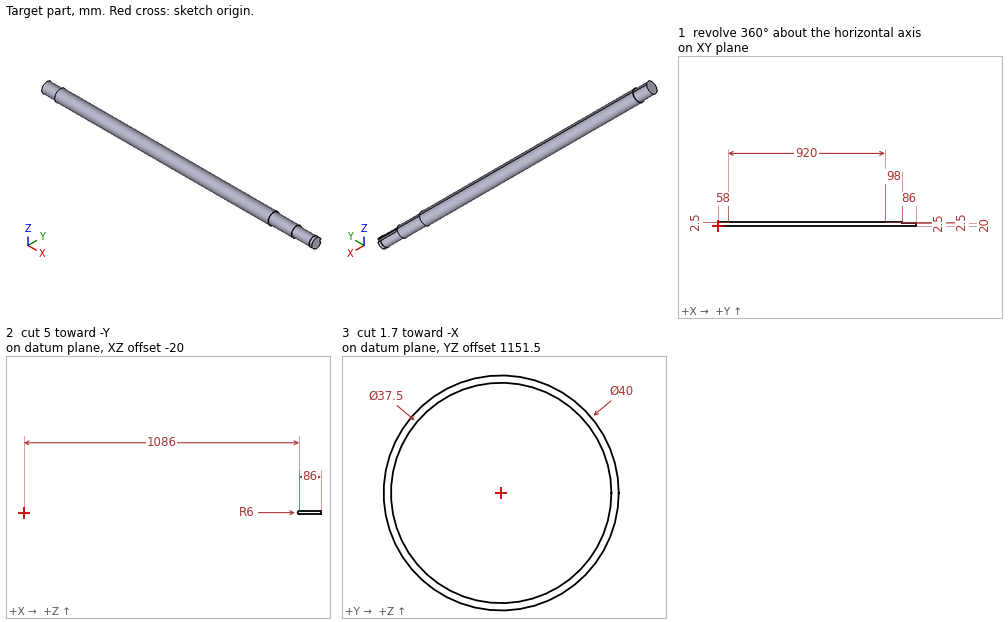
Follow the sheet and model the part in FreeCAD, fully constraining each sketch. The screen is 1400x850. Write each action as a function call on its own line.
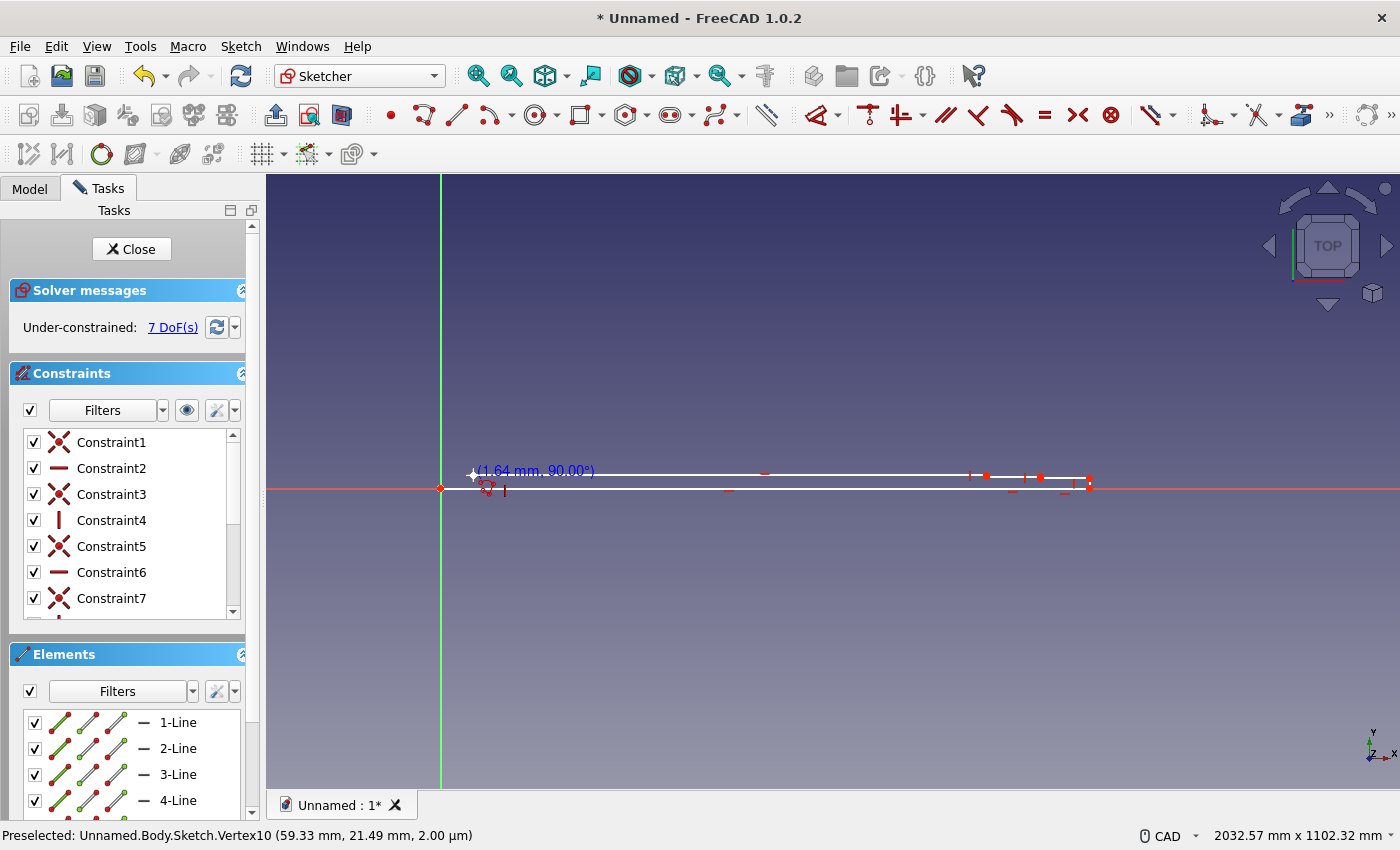
scroll(473, 476, up, 13)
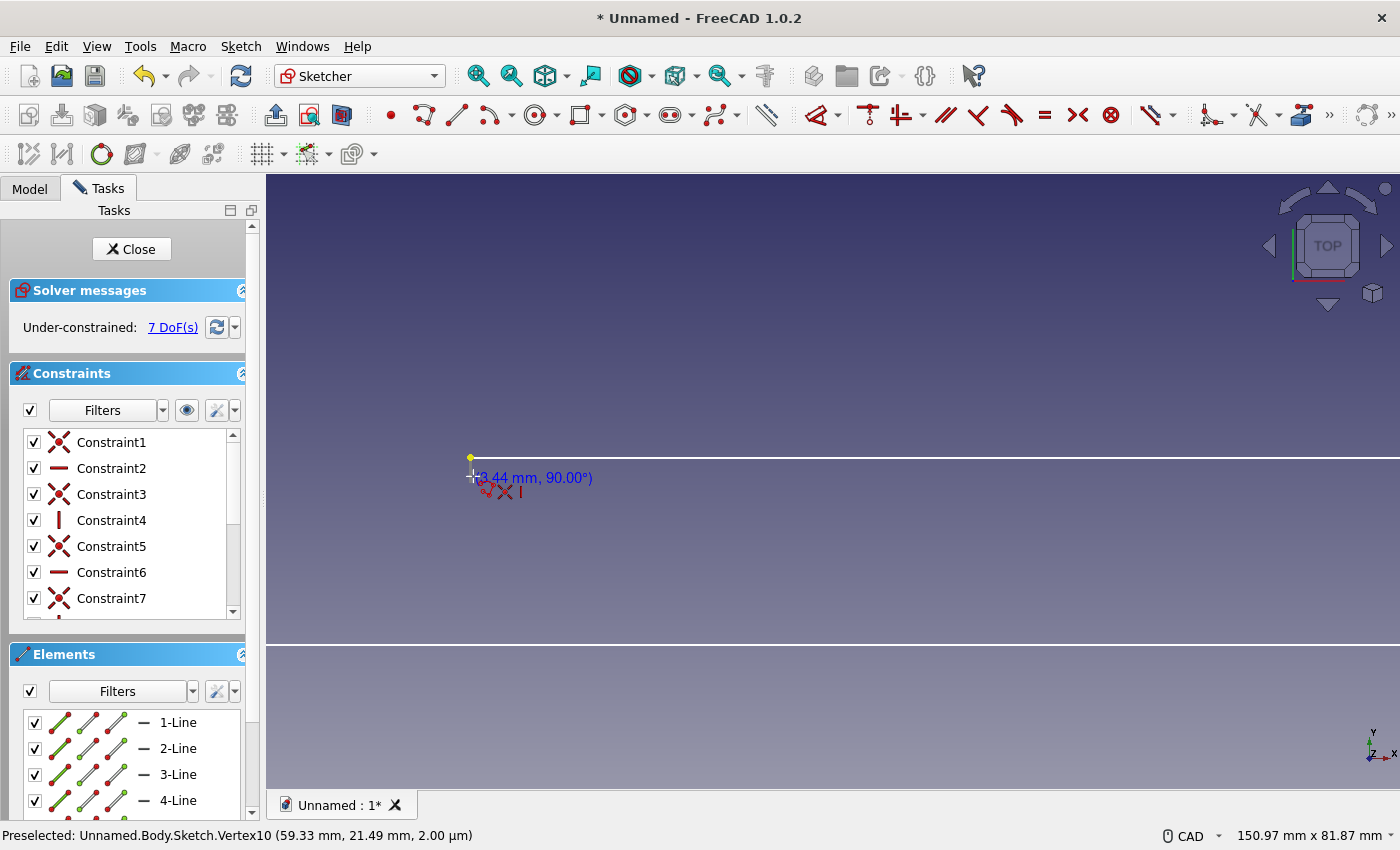
click(471, 476)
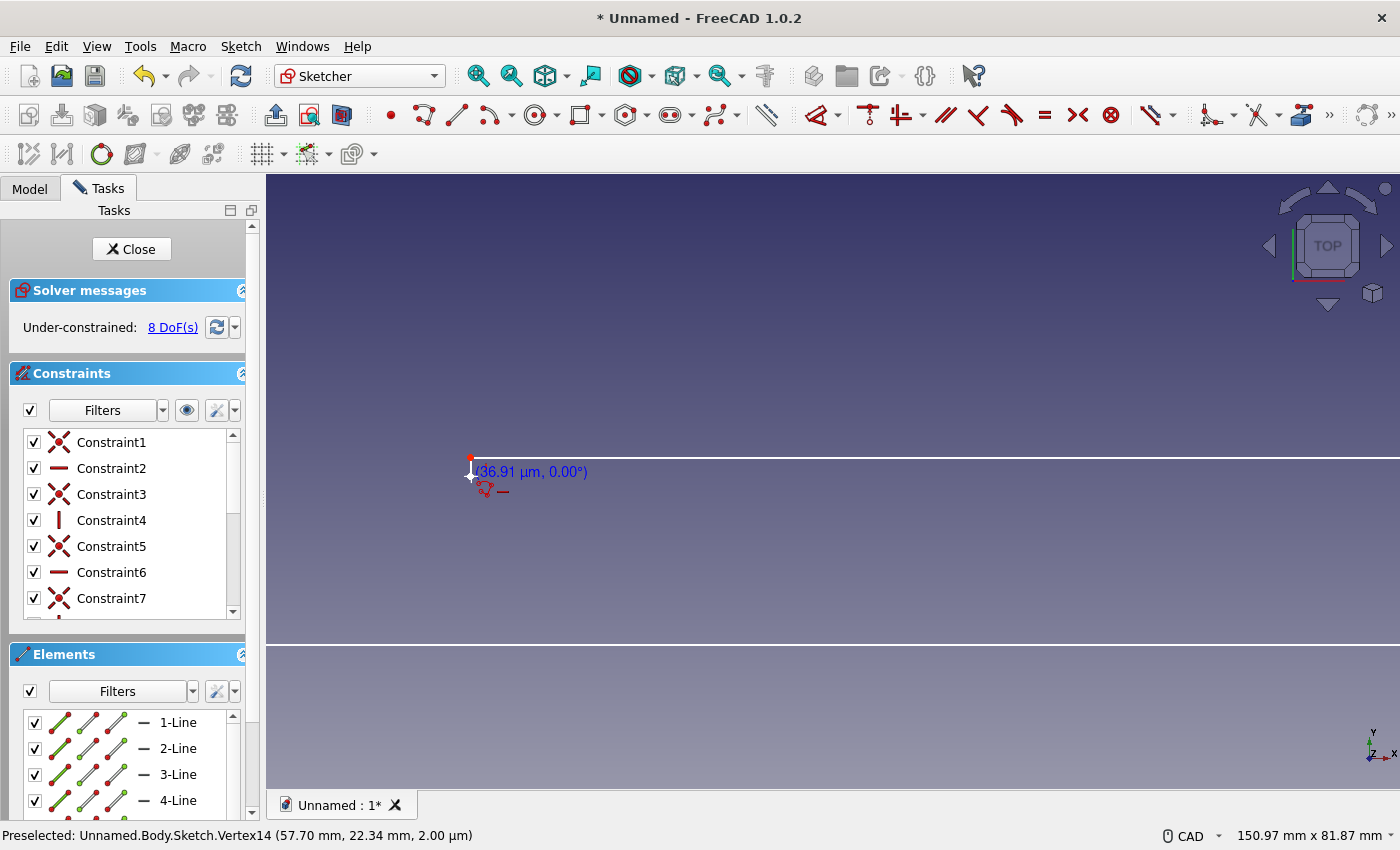
scroll(473, 476, down, 13)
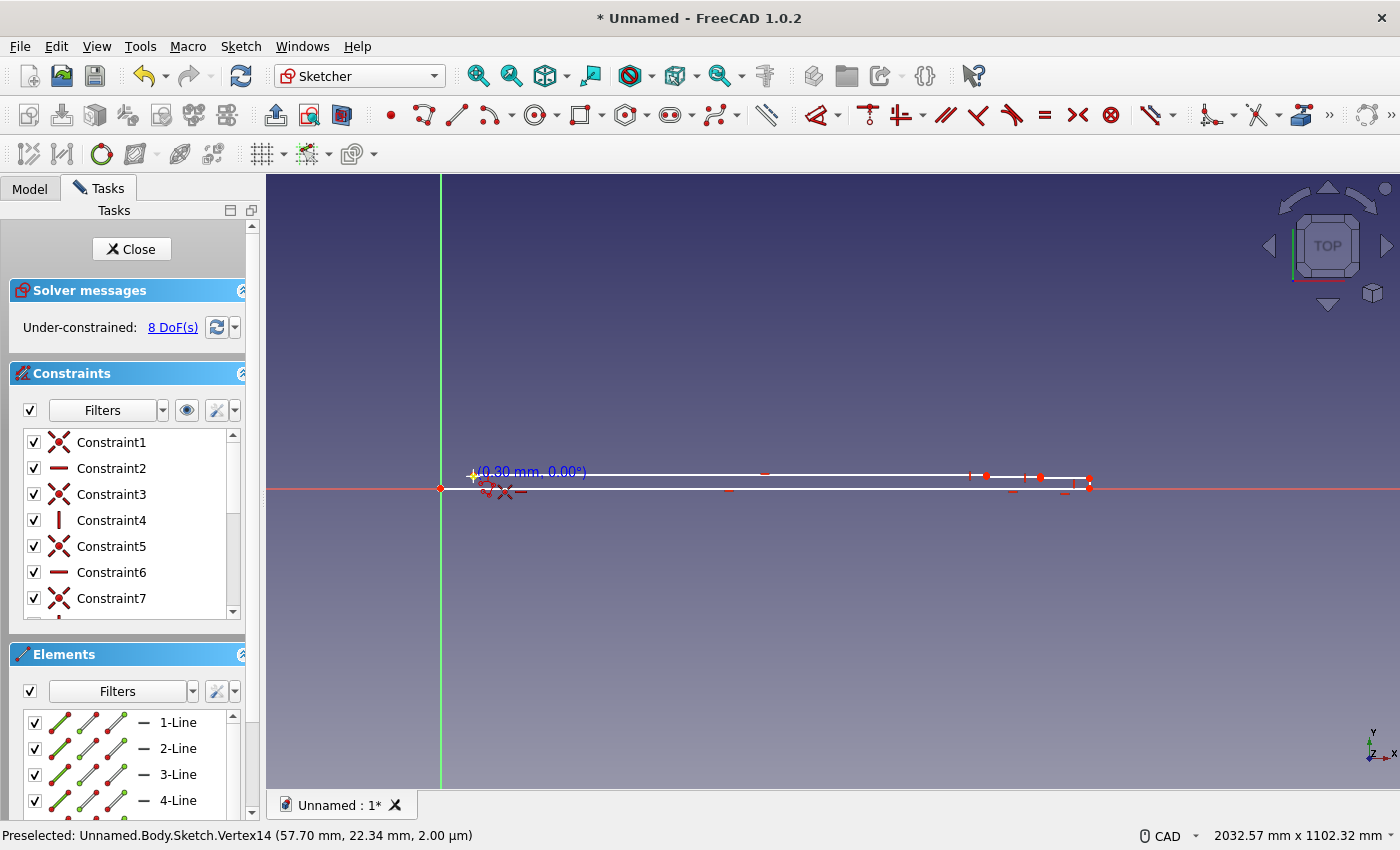
scroll(441, 476, up, 2)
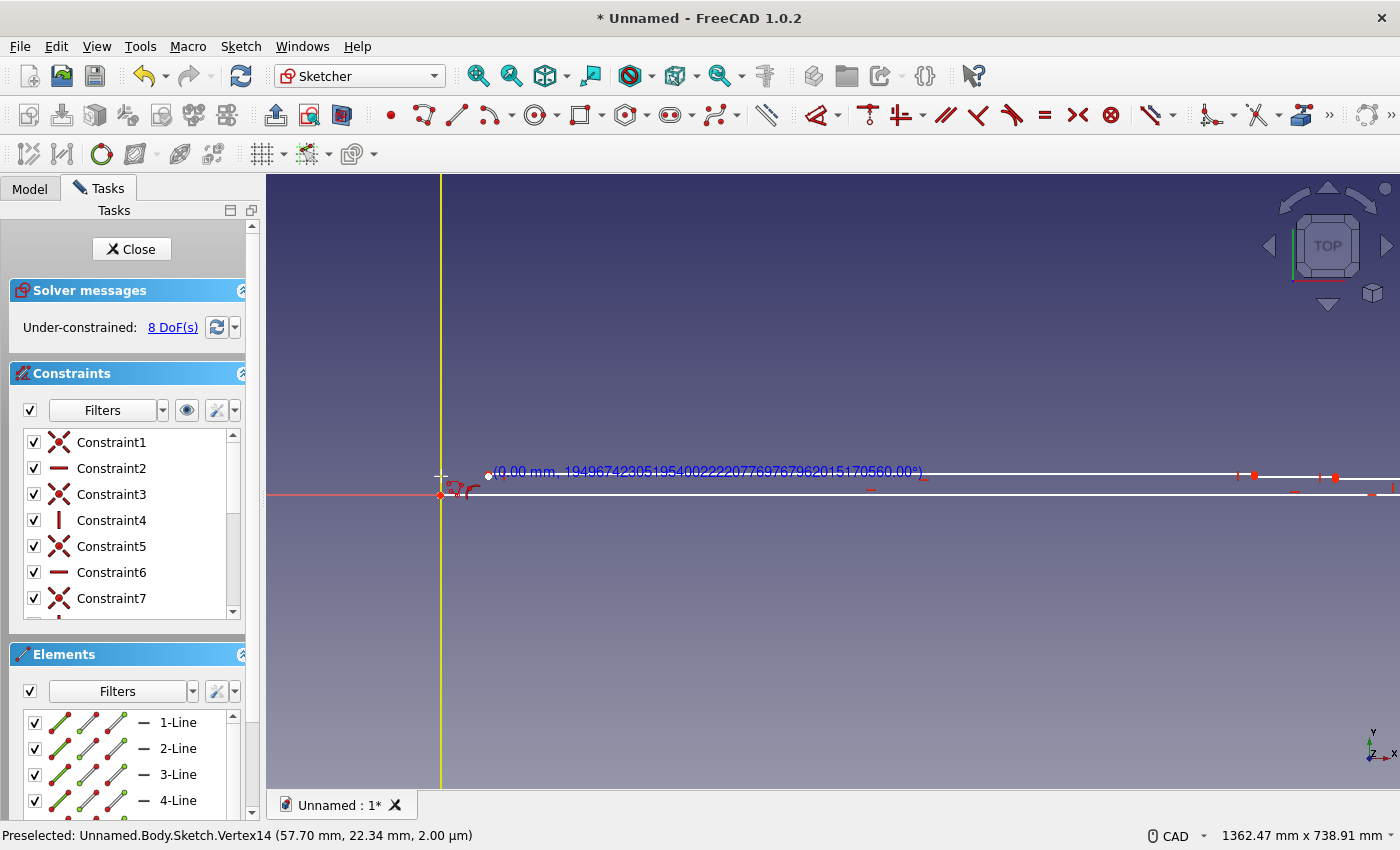
click(450, 476)
click(441, 495)
key(Escape)
key(Escape)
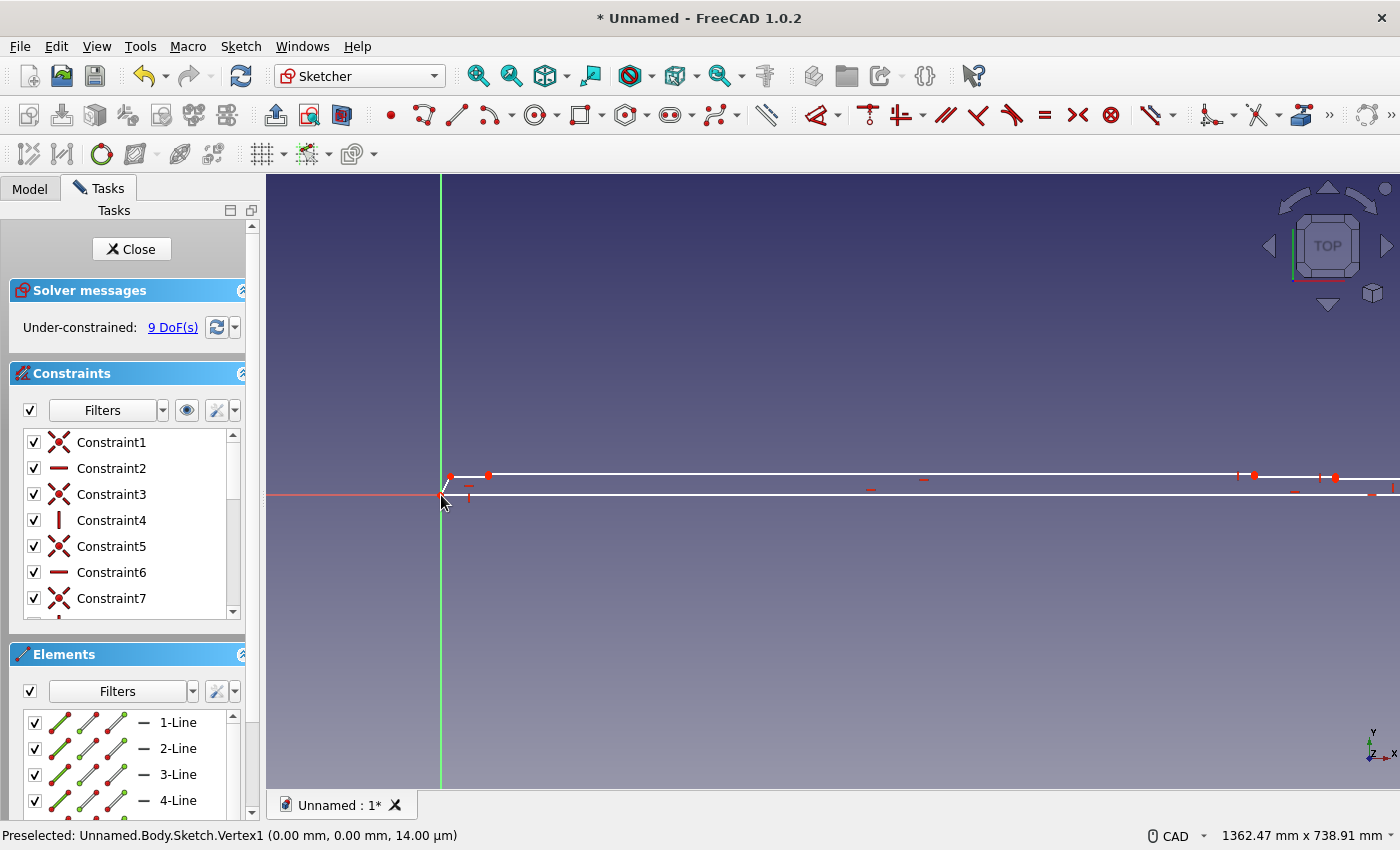
scroll(444, 488, up, 4)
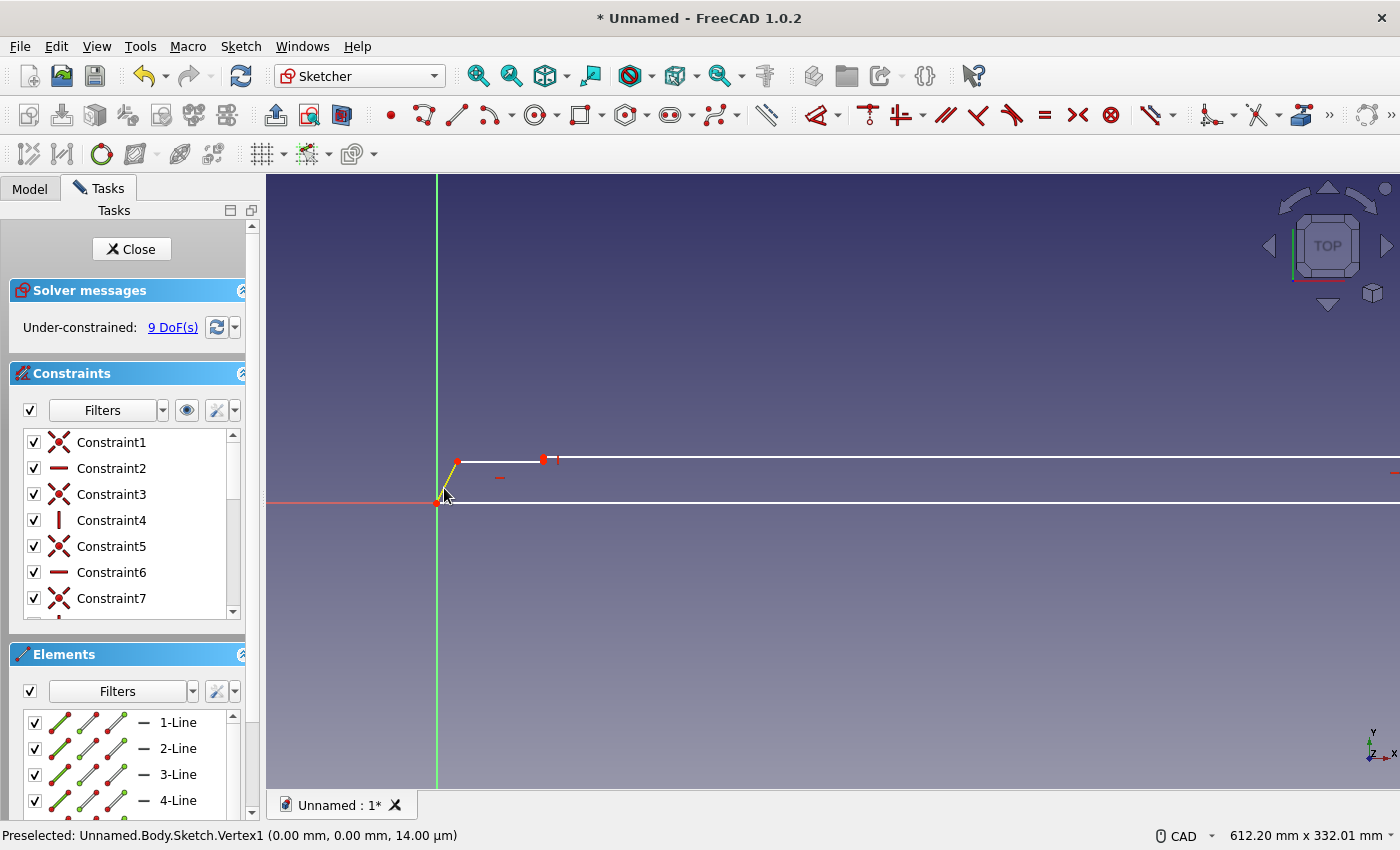
click(445, 487)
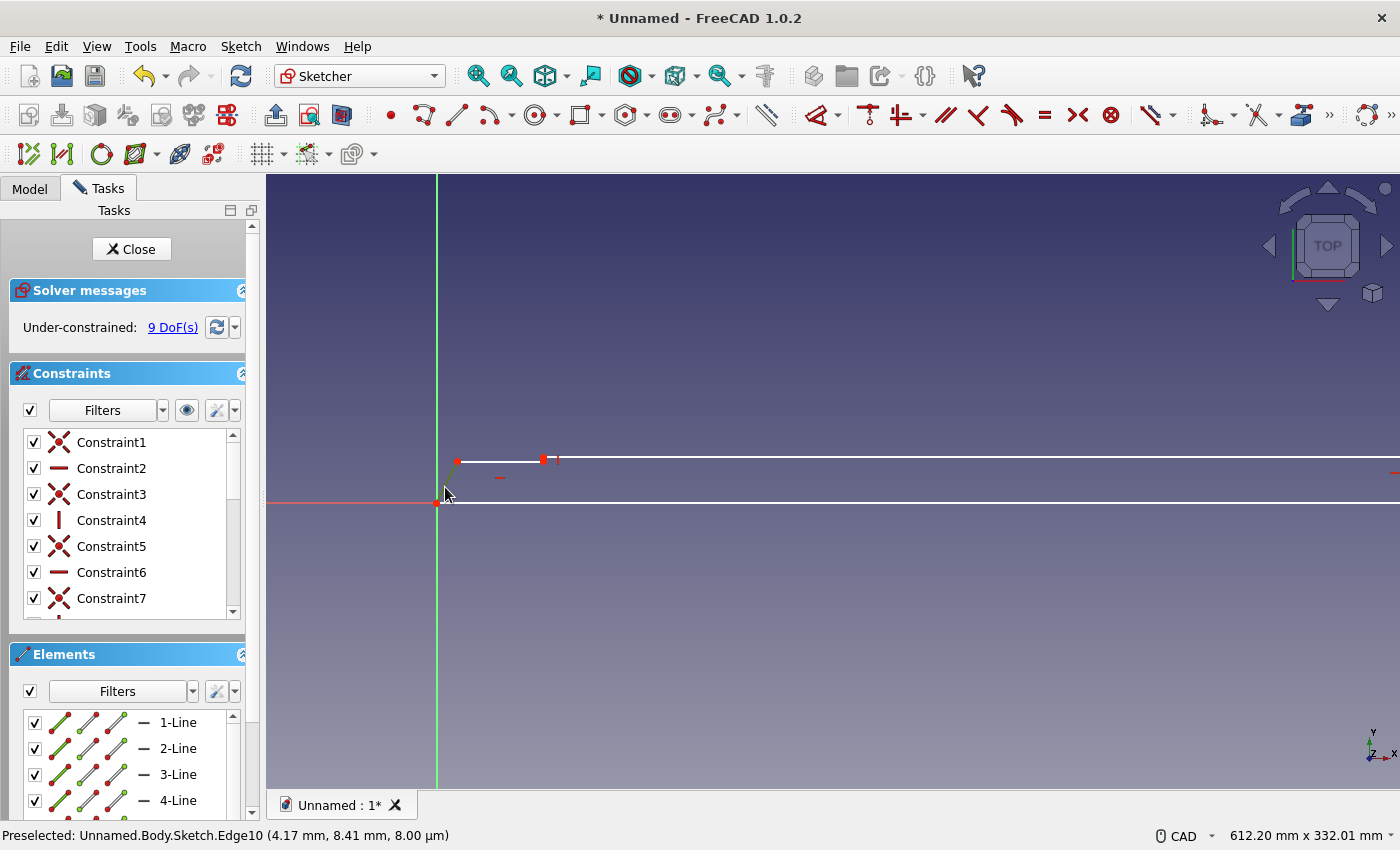
click(922, 116)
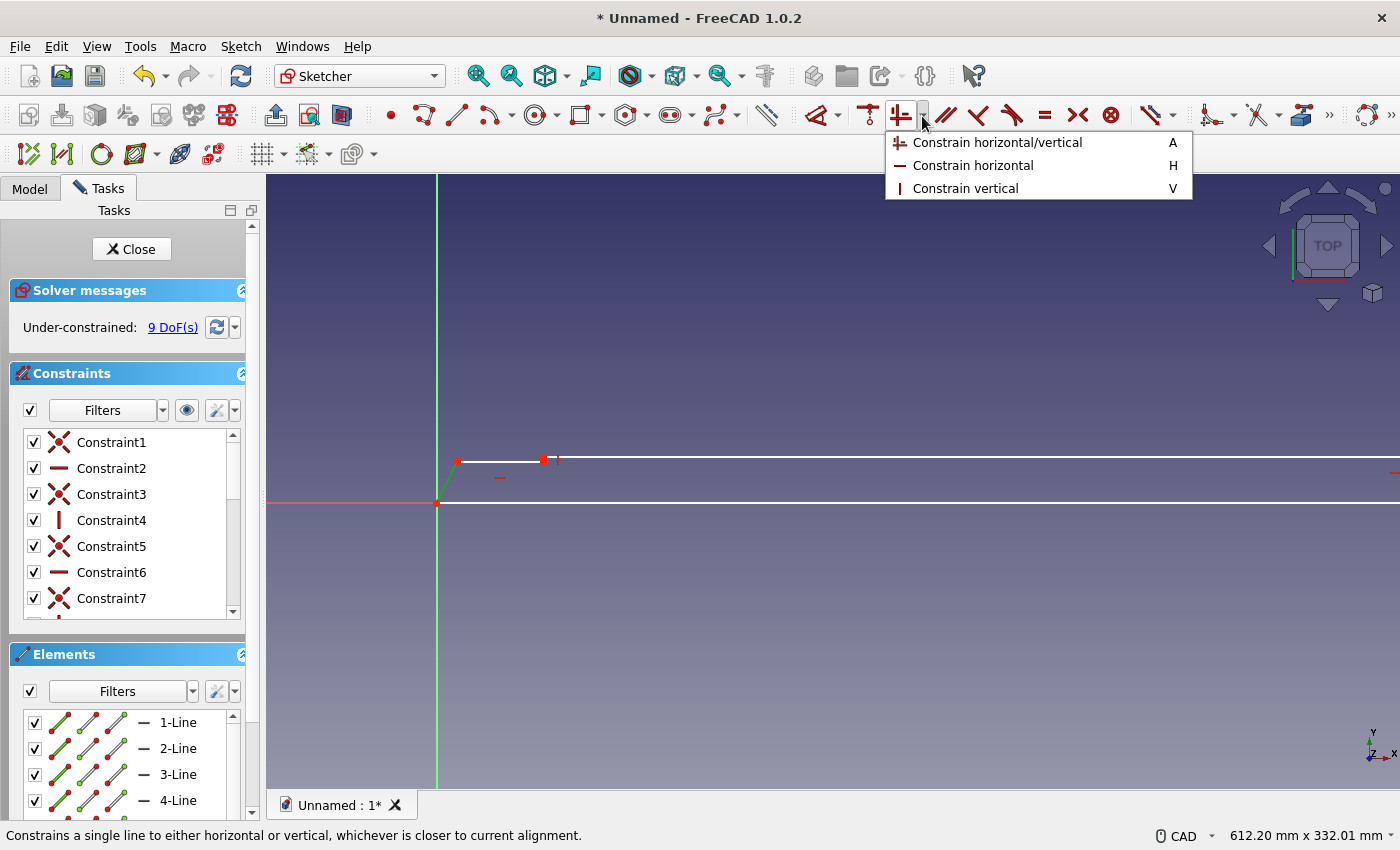
click(1039, 188)